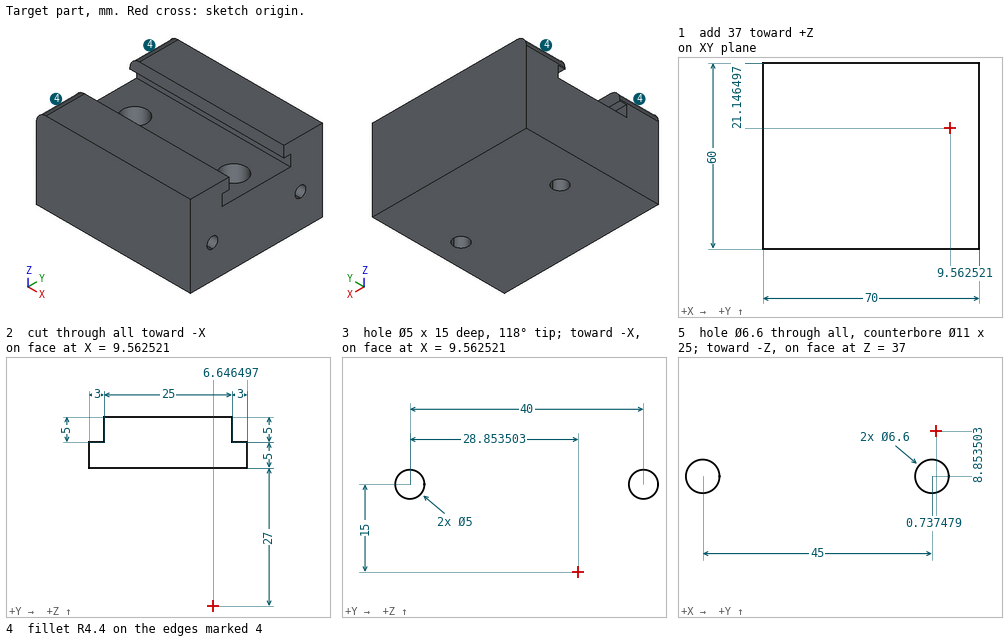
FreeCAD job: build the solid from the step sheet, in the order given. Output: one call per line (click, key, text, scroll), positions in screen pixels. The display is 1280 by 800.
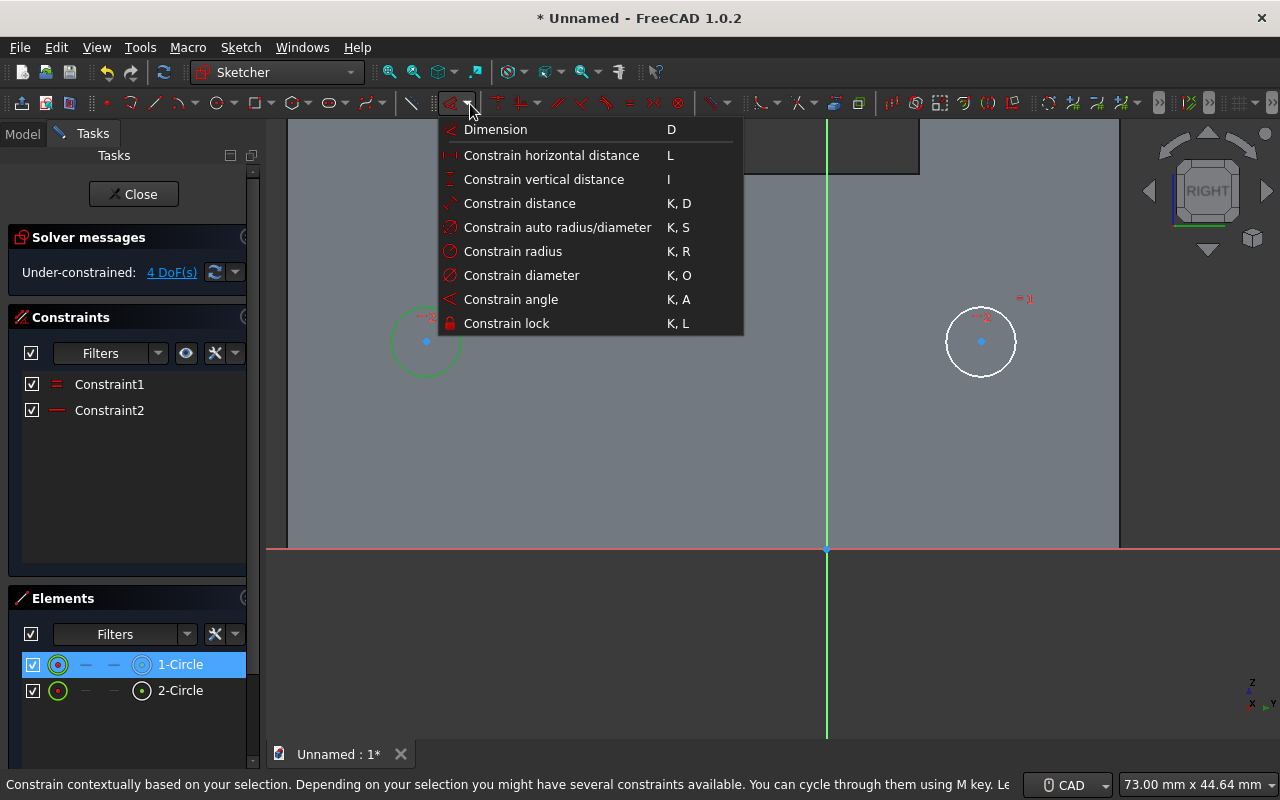
click(591, 275)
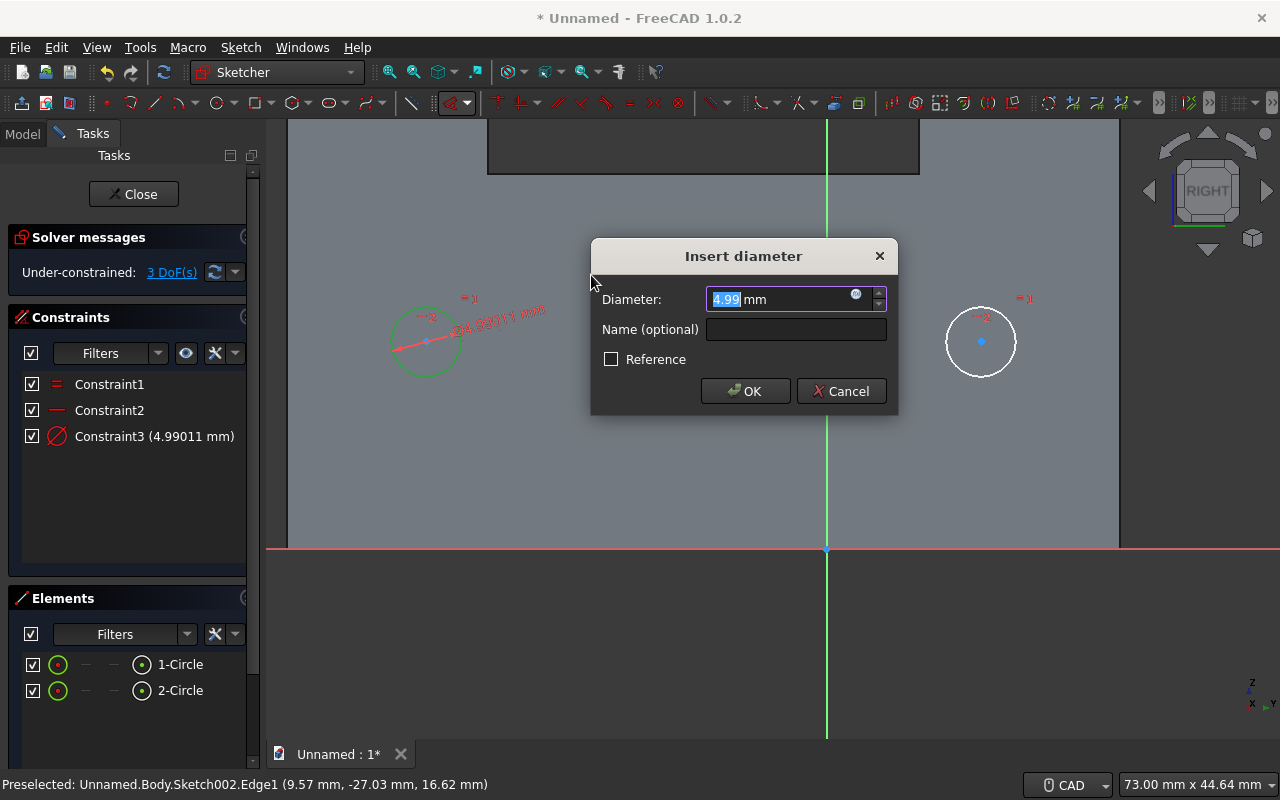
text(5)
key(Return)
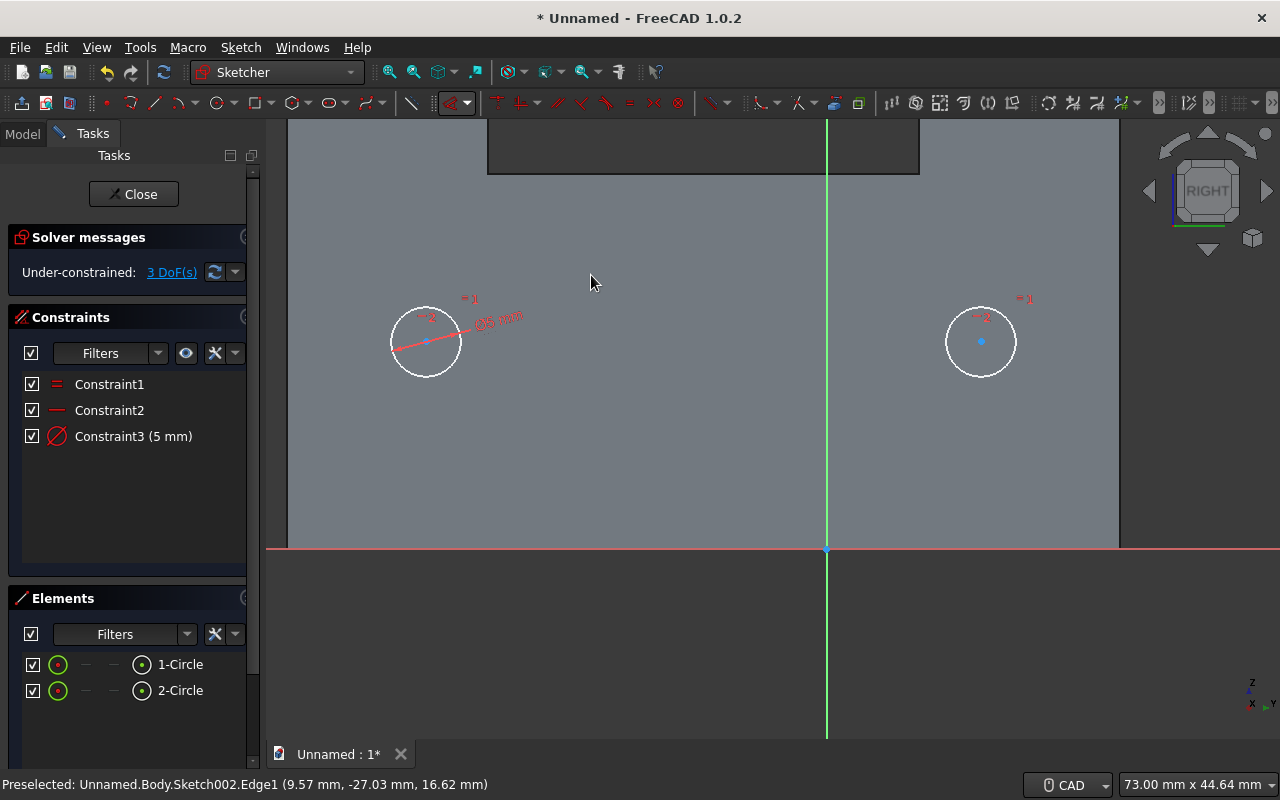
click(426, 342)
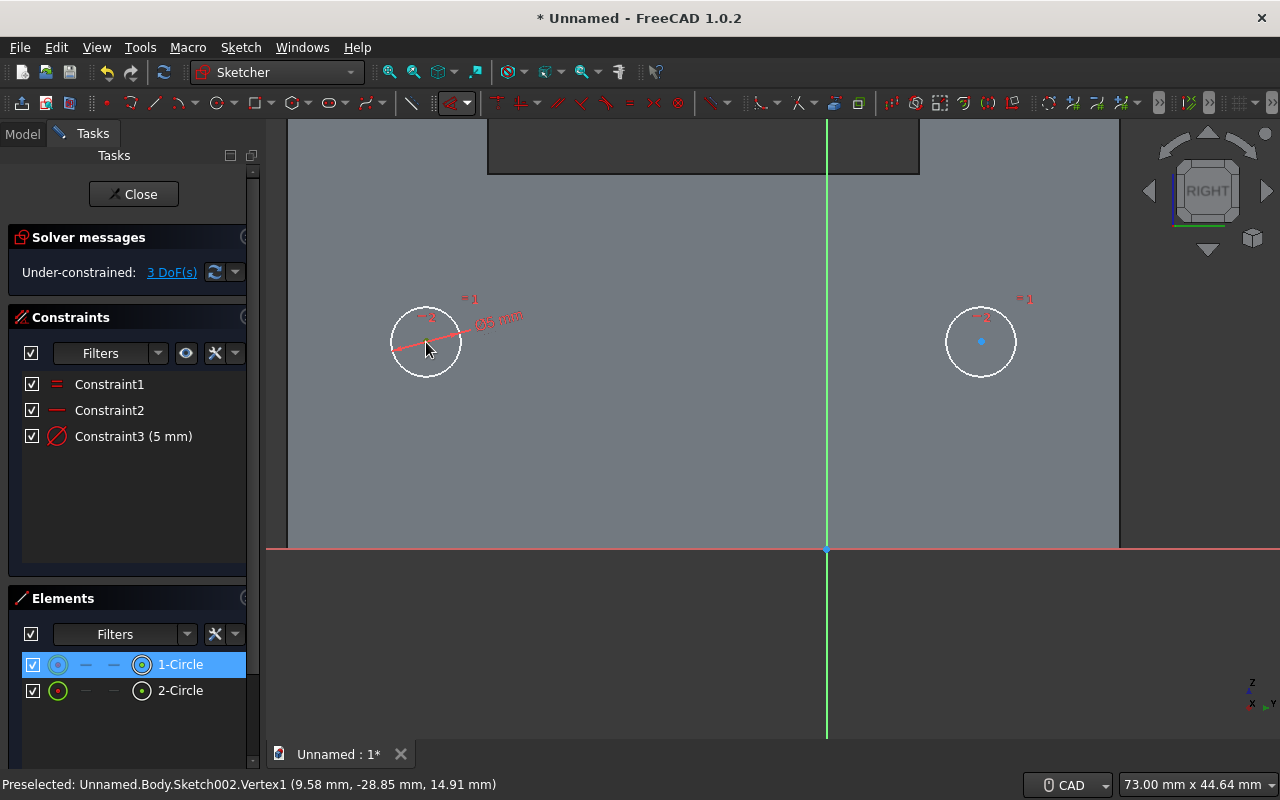
click(470, 104)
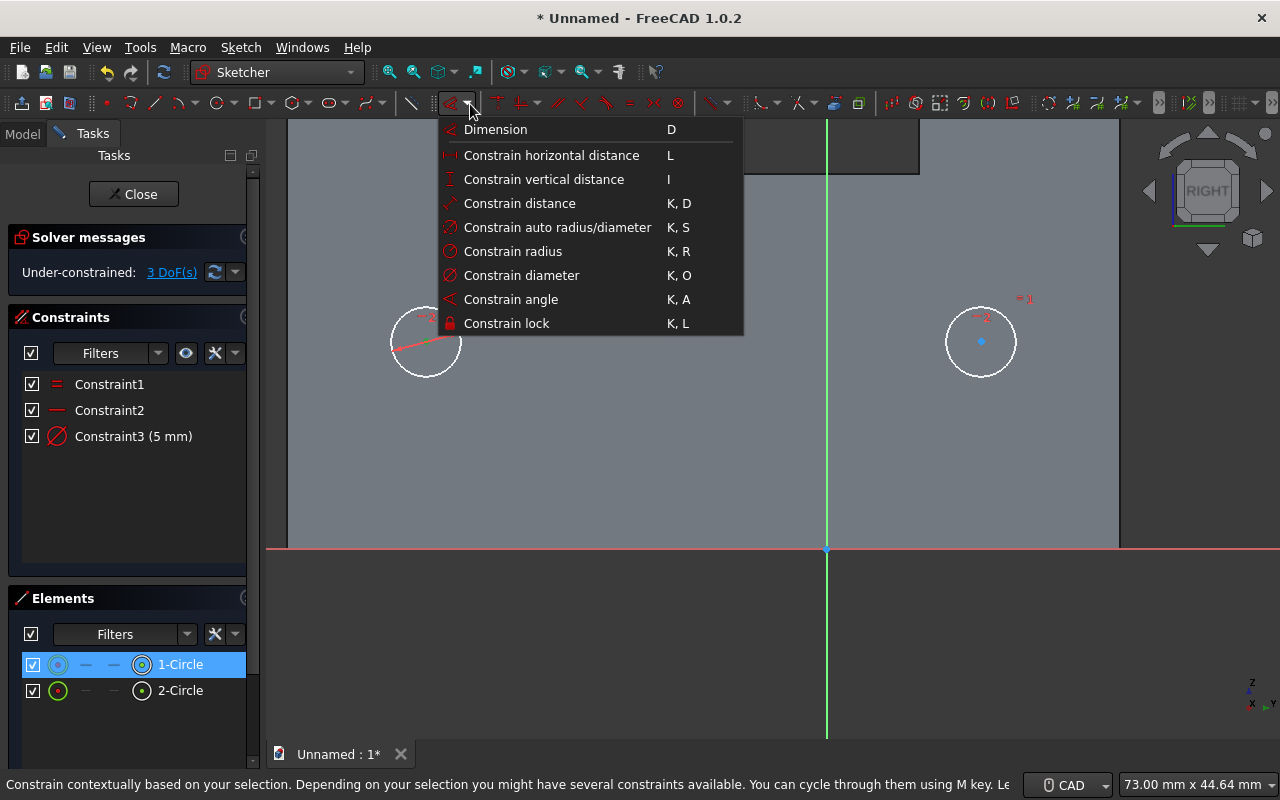
click(591, 179)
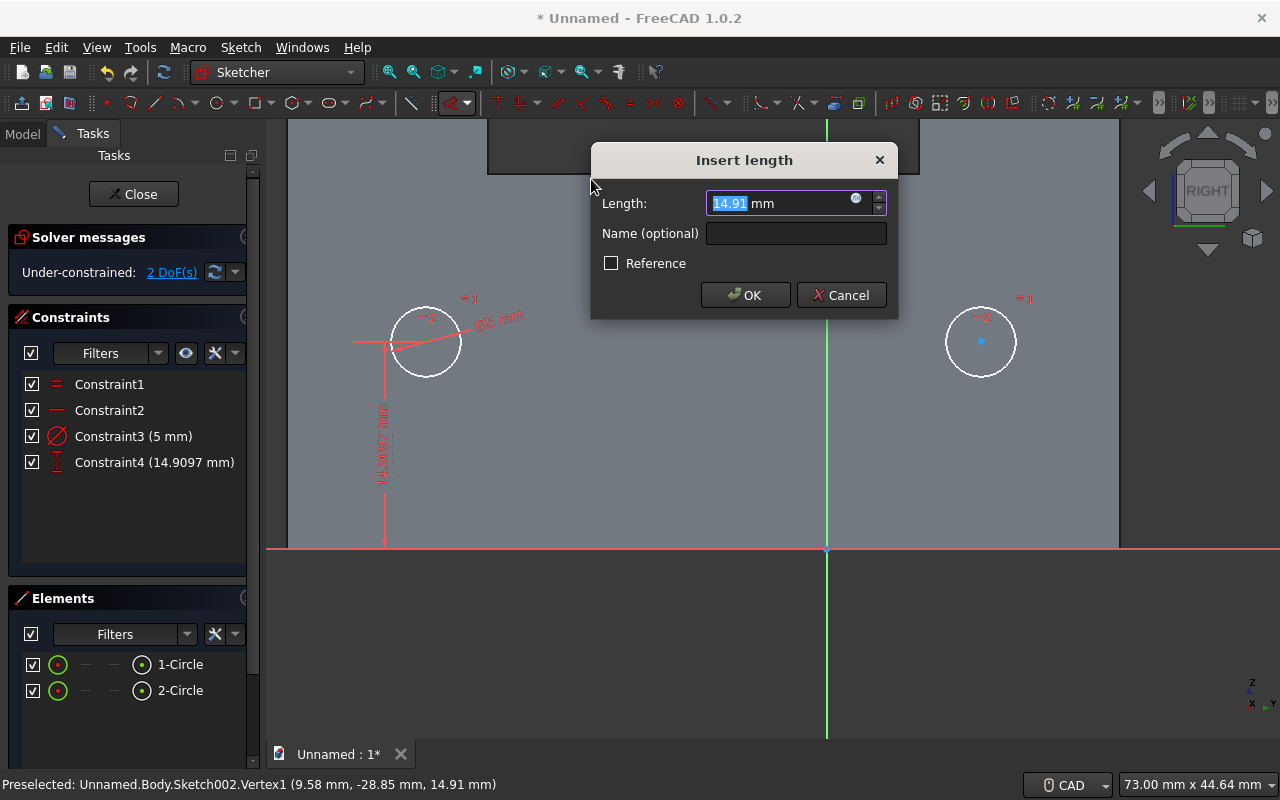
text(15)
key(Return)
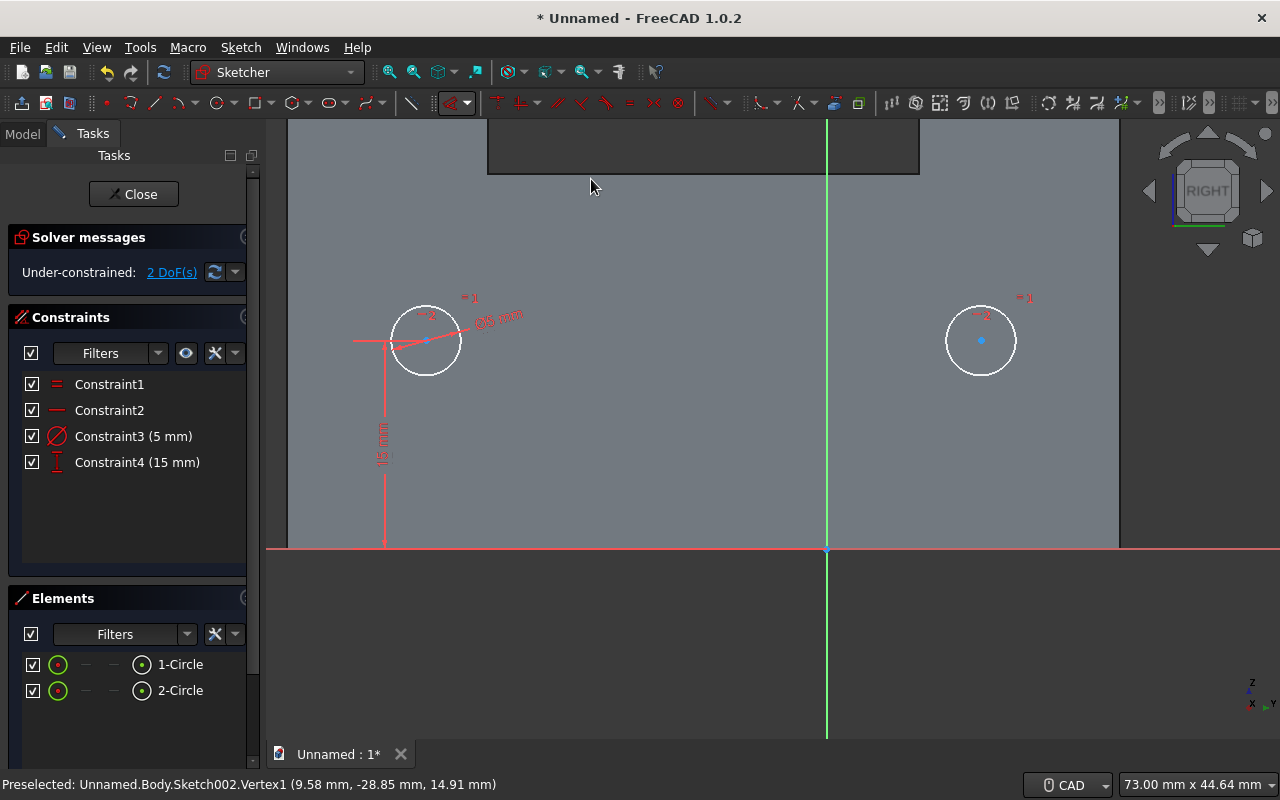
click(426, 341)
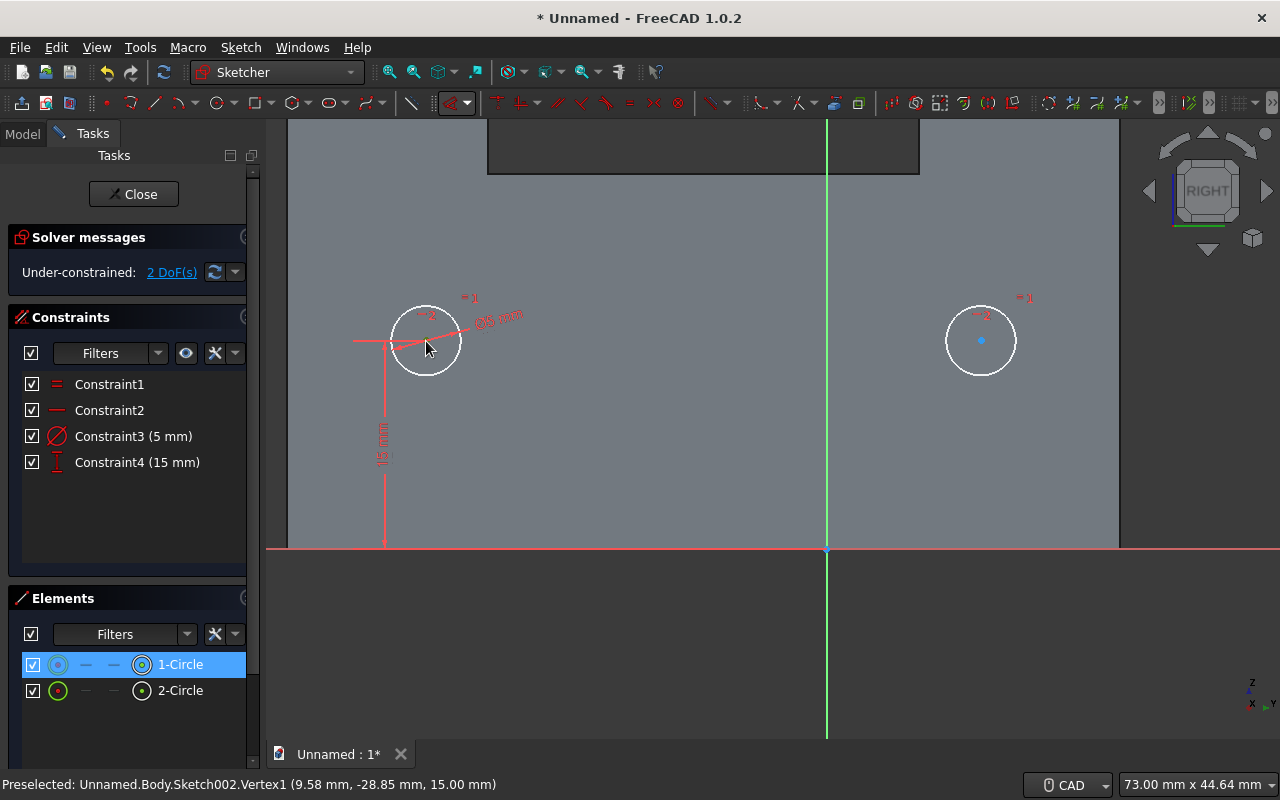
click(981, 341)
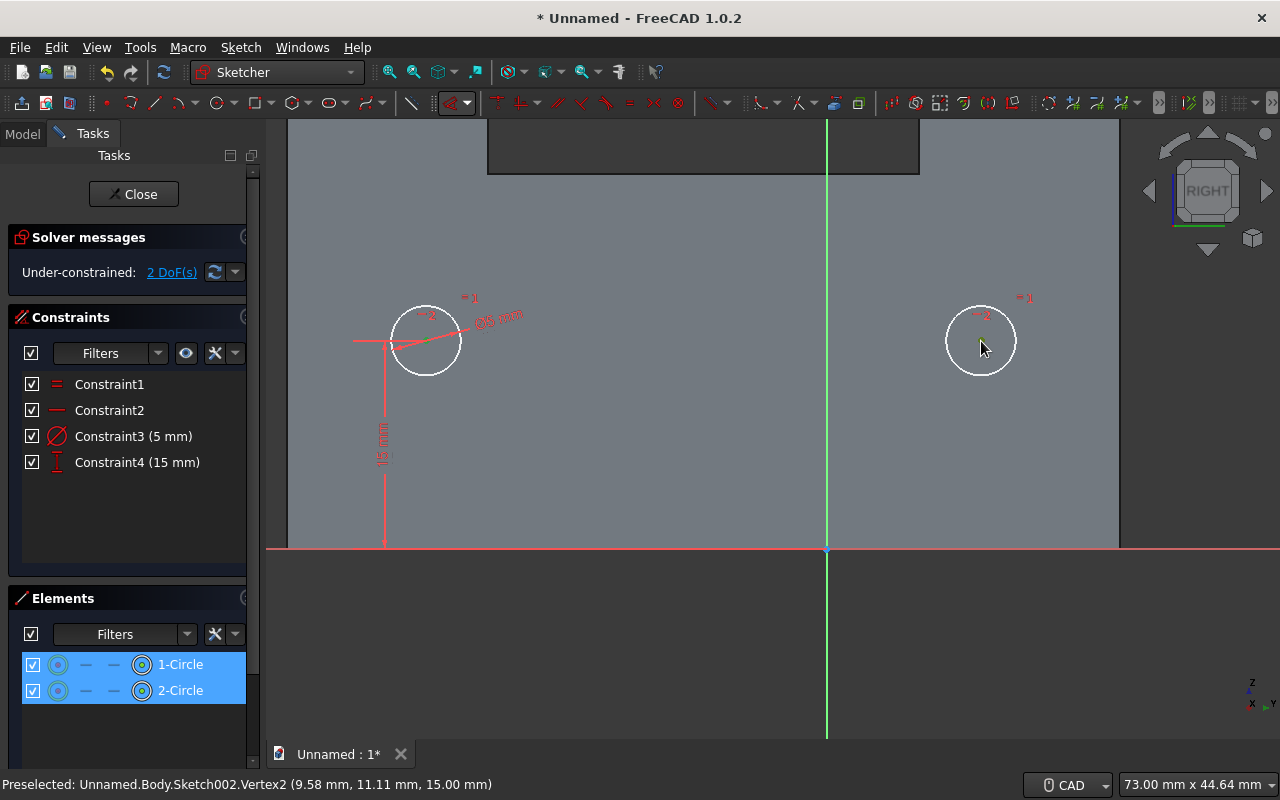
key(l)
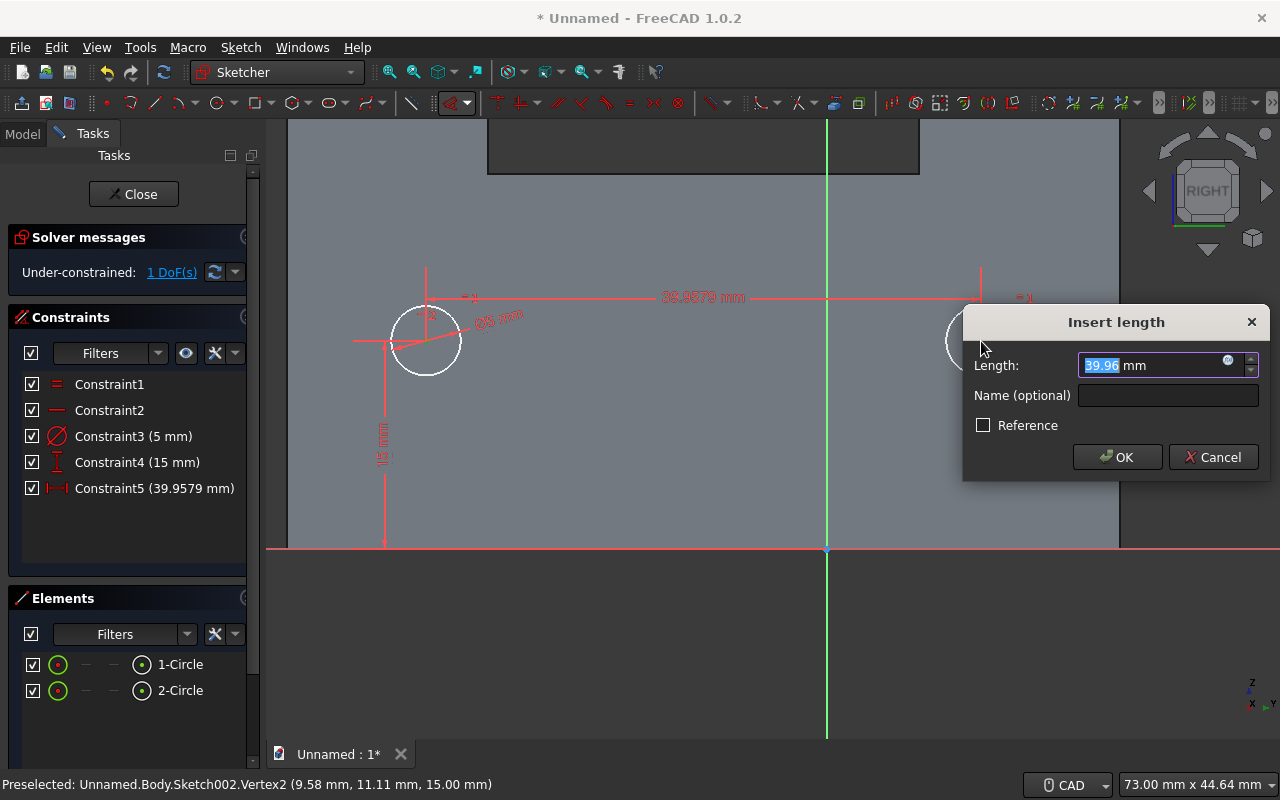
text(40)
key(Return)